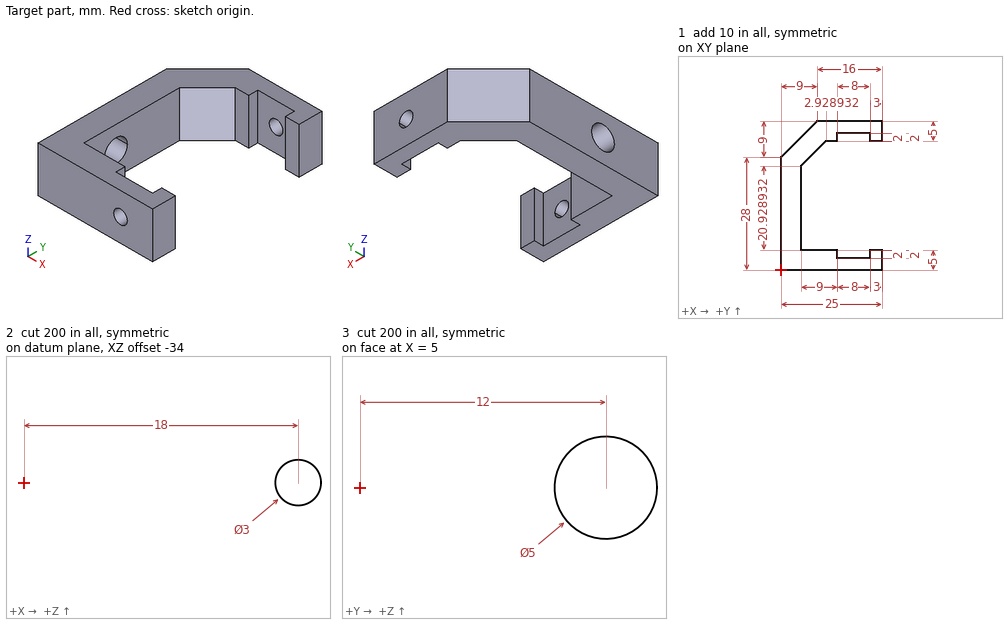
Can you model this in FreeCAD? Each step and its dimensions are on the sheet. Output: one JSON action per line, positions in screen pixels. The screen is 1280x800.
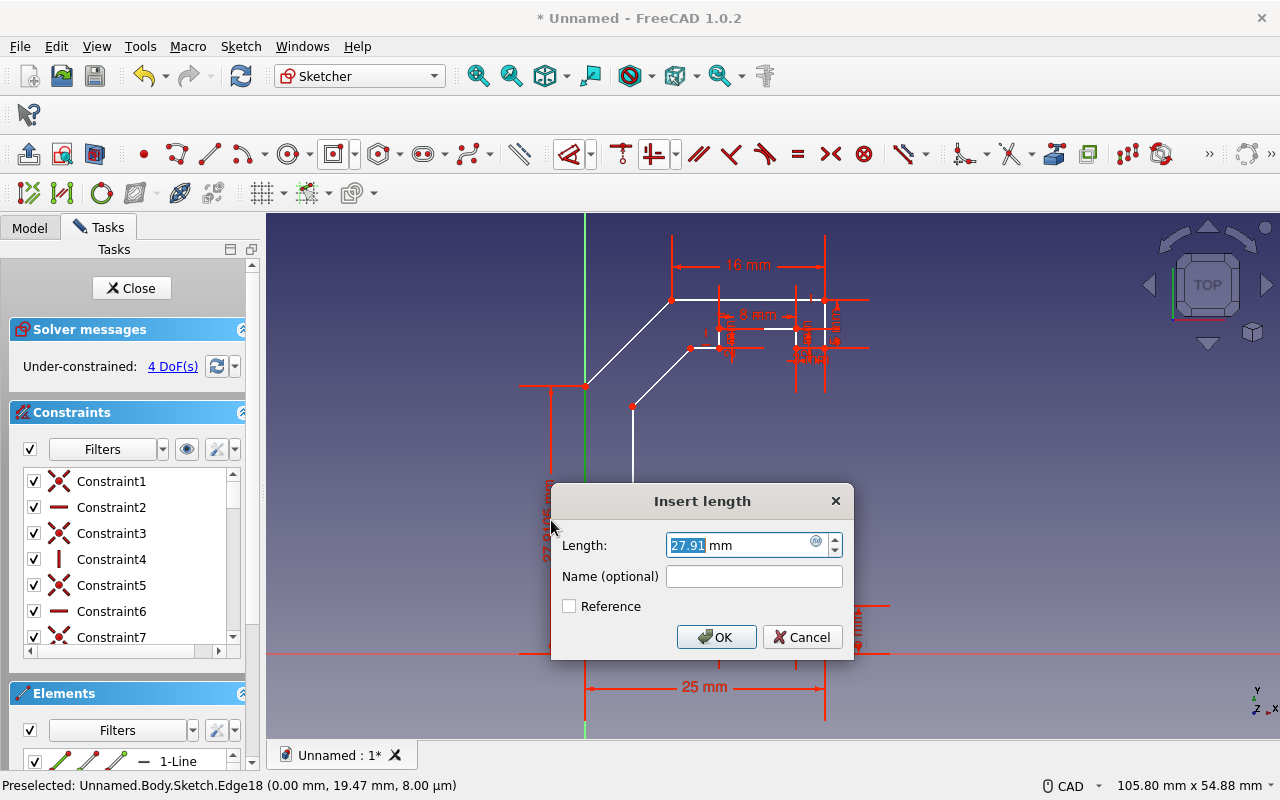
{"action": "type", "text": "28"}
{"action": "key", "text": "Return"}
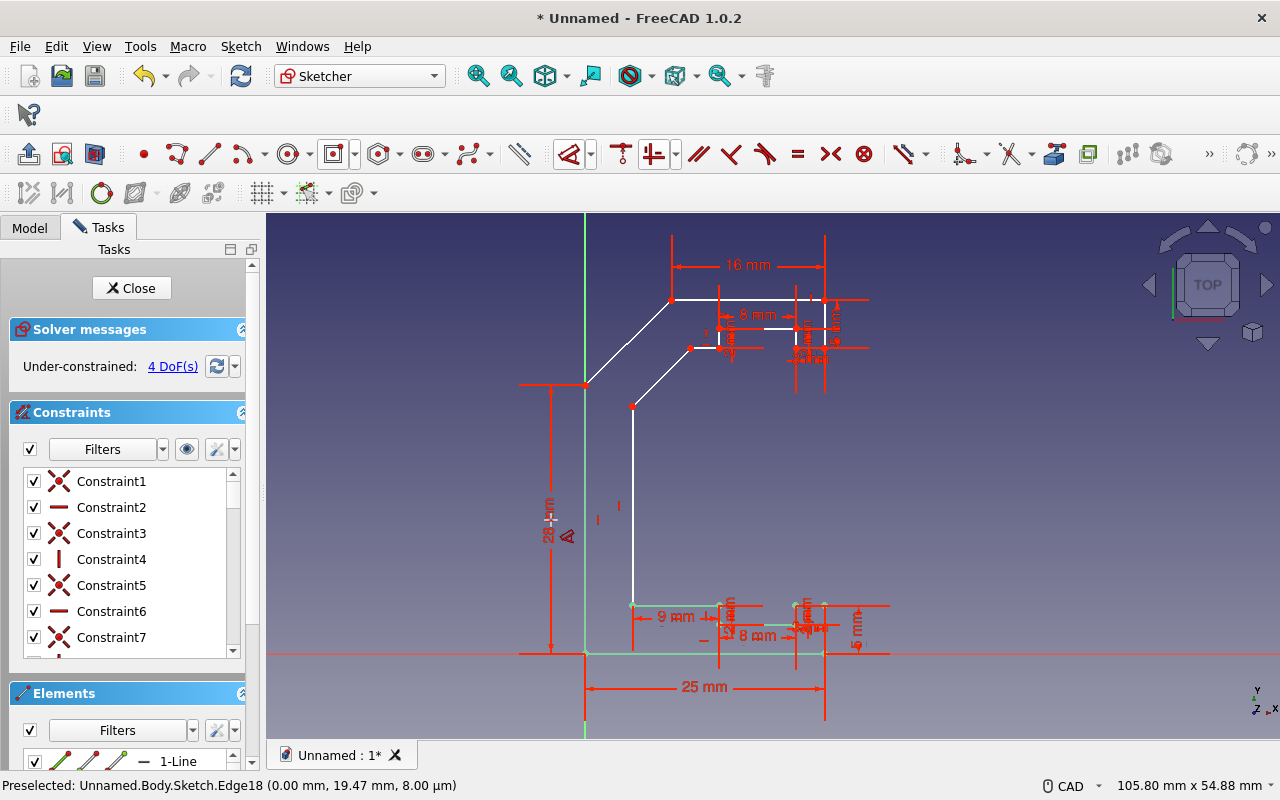
{"action": "left_click", "coordinate": [672, 300]}
{"action": "left_click", "coordinate": [628, 688]}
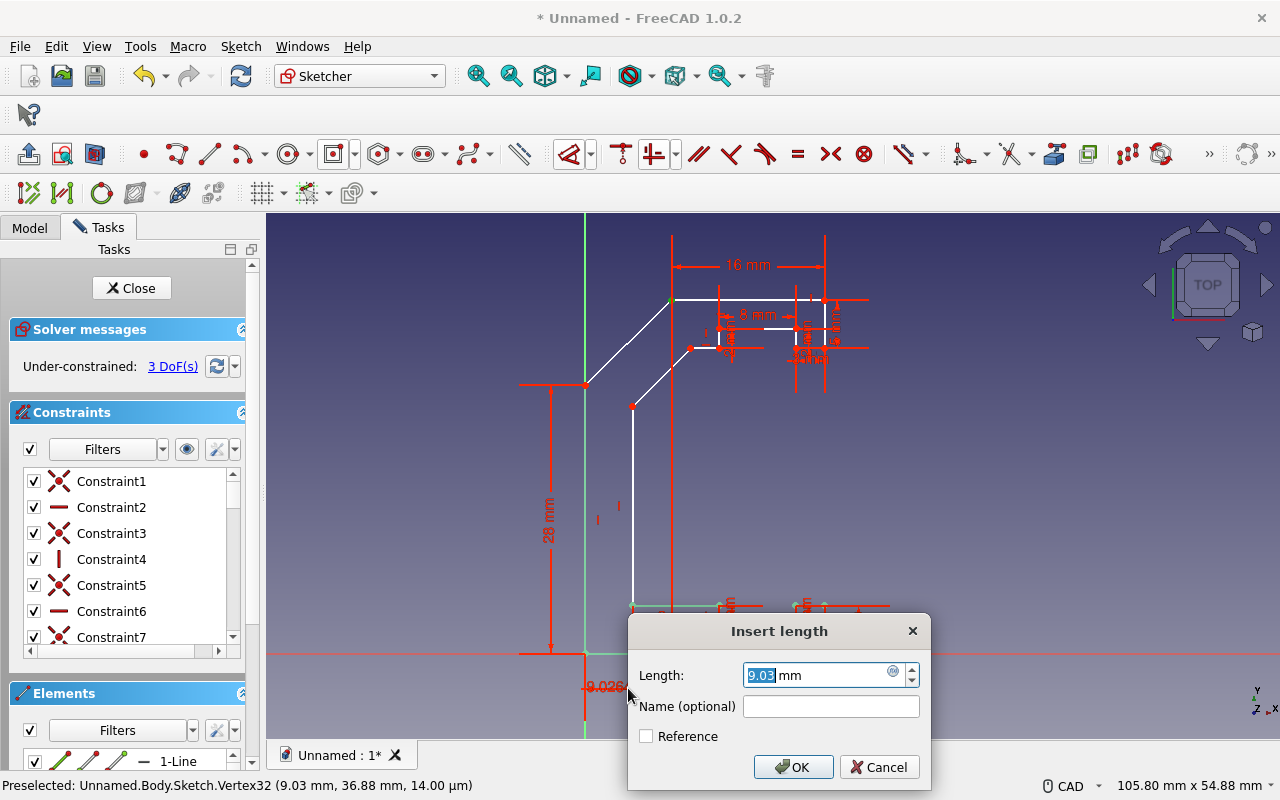
{"action": "type", "text": "9"}
{"action": "key", "text": "Return"}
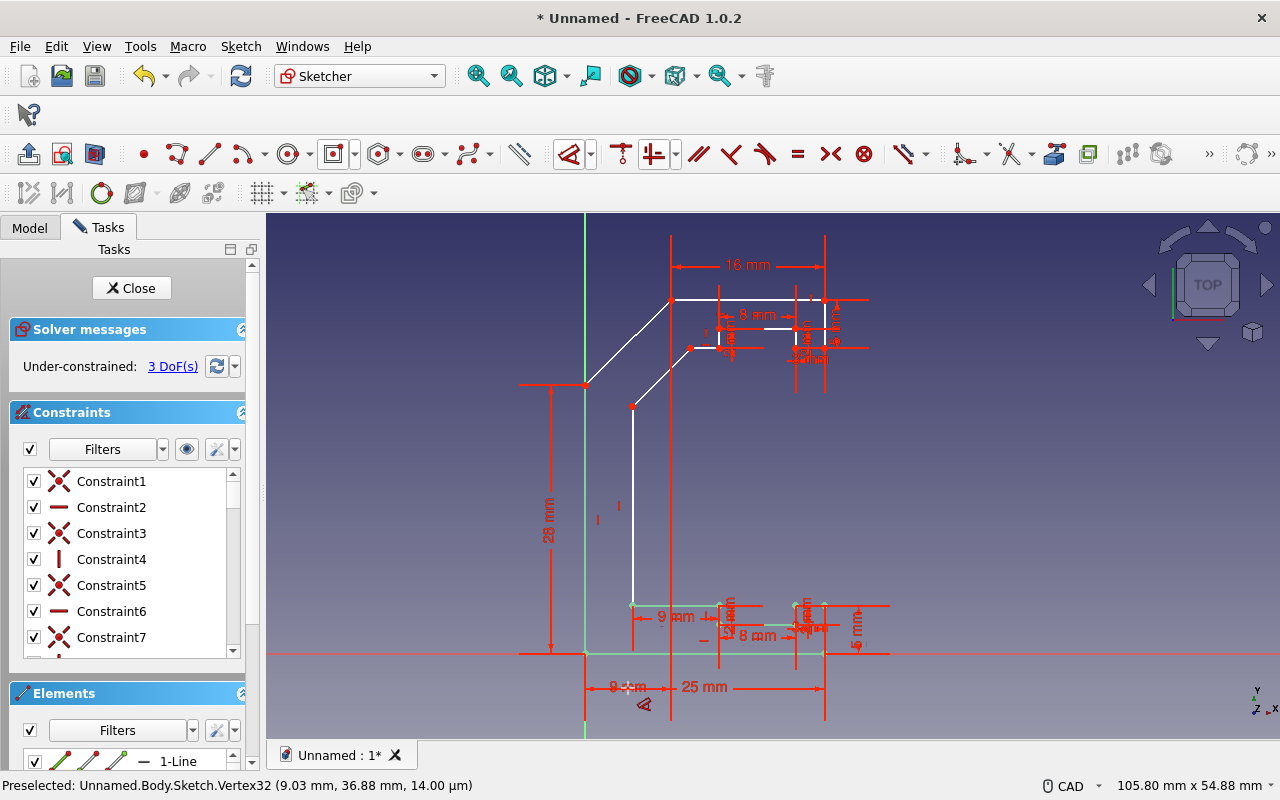
{"action": "left_click", "coordinate": [645, 326]}
{"action": "left_click", "coordinate": [551, 343]}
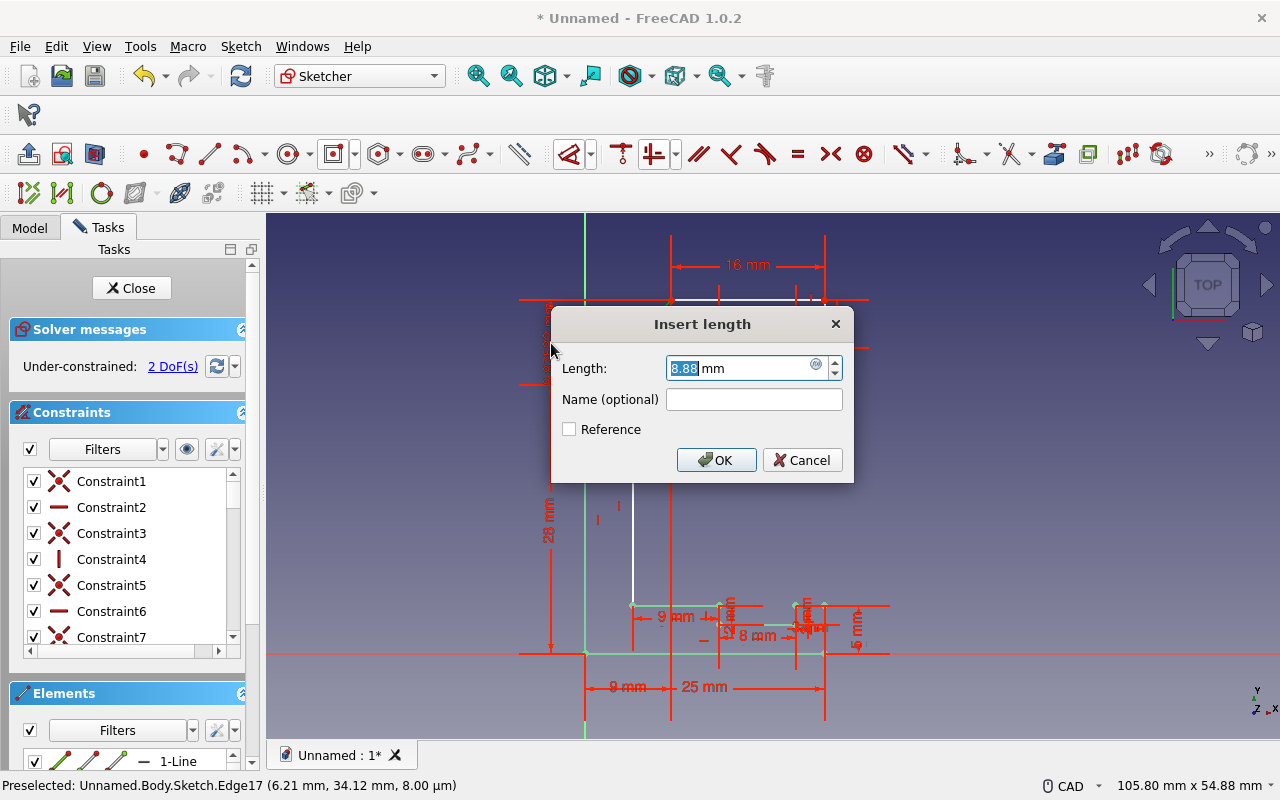
{"action": "type", "text": "9"}
{"action": "key", "text": "Return"}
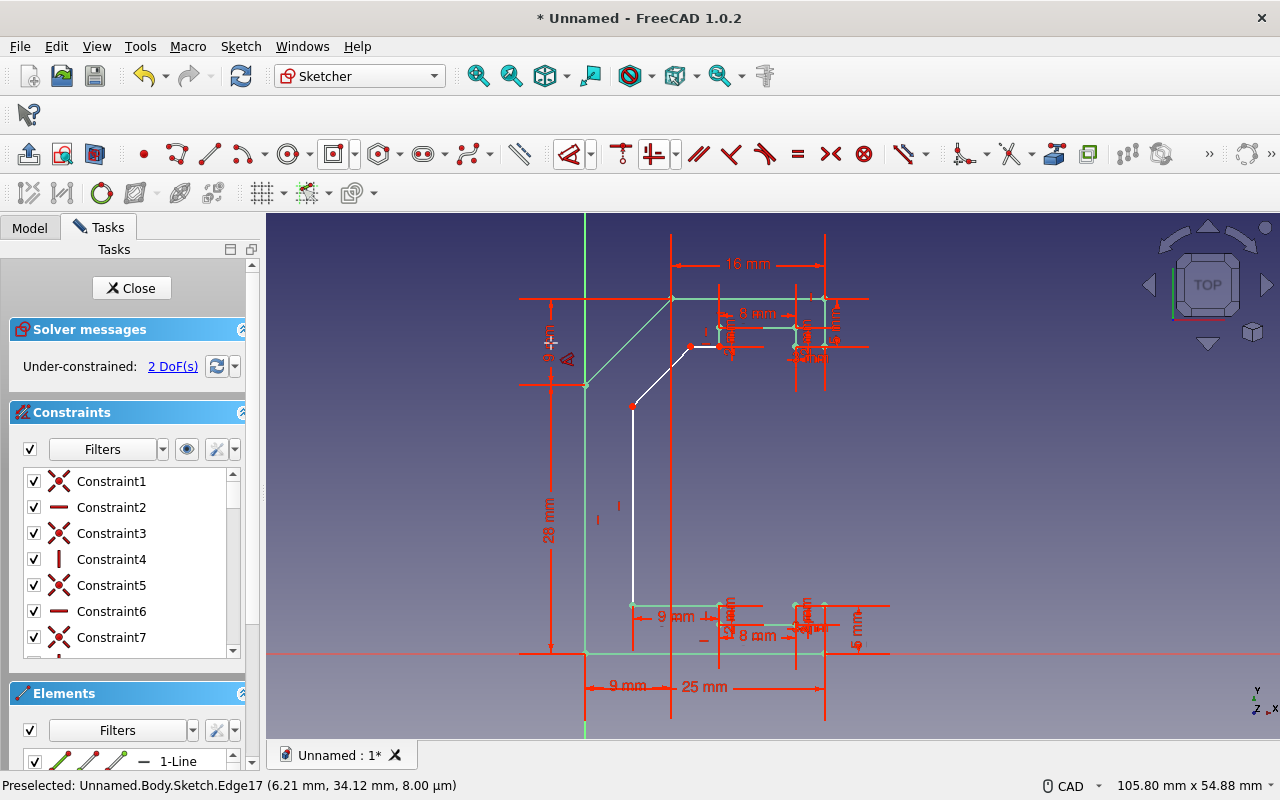
{"action": "scroll", "coordinate": [702, 347], "scroll_direction": "up", "scroll_amount": 2}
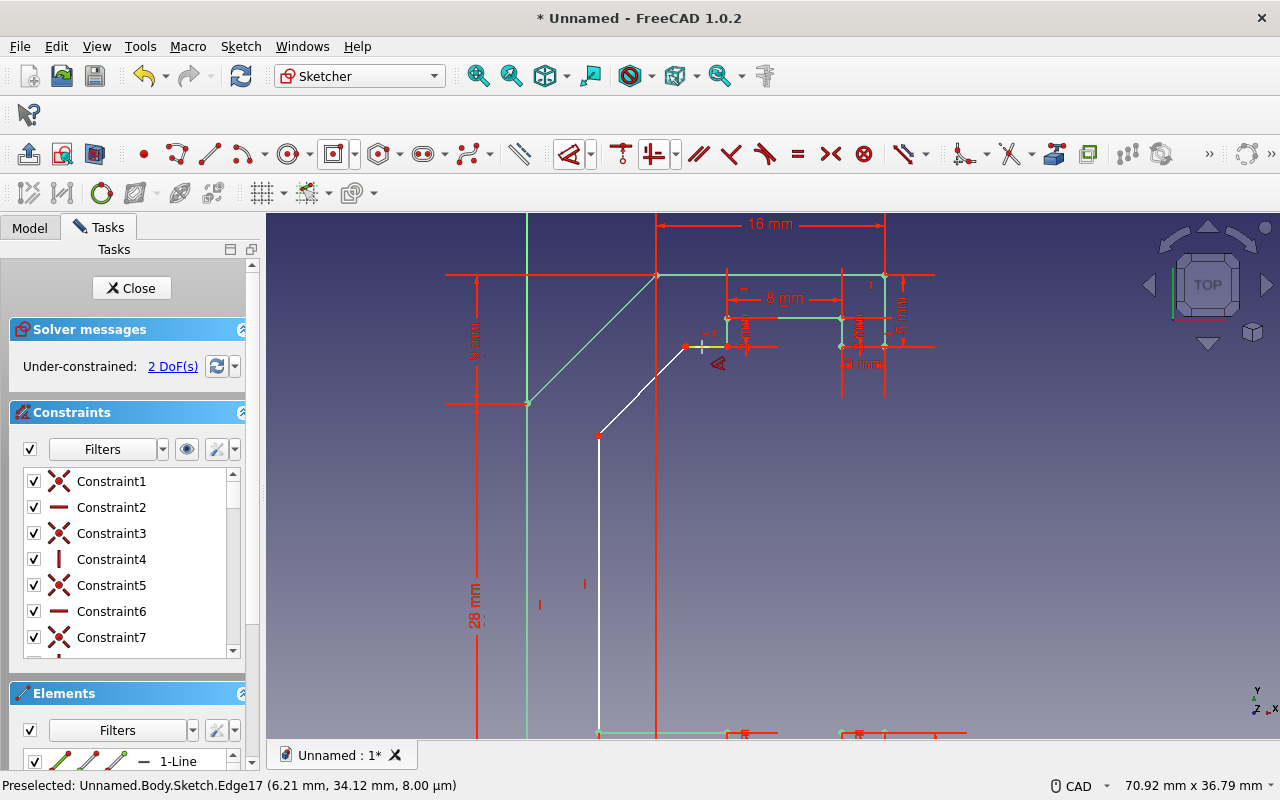
{"action": "left_click", "coordinate": [702, 347]}
{"action": "left_click", "coordinate": [706, 313]}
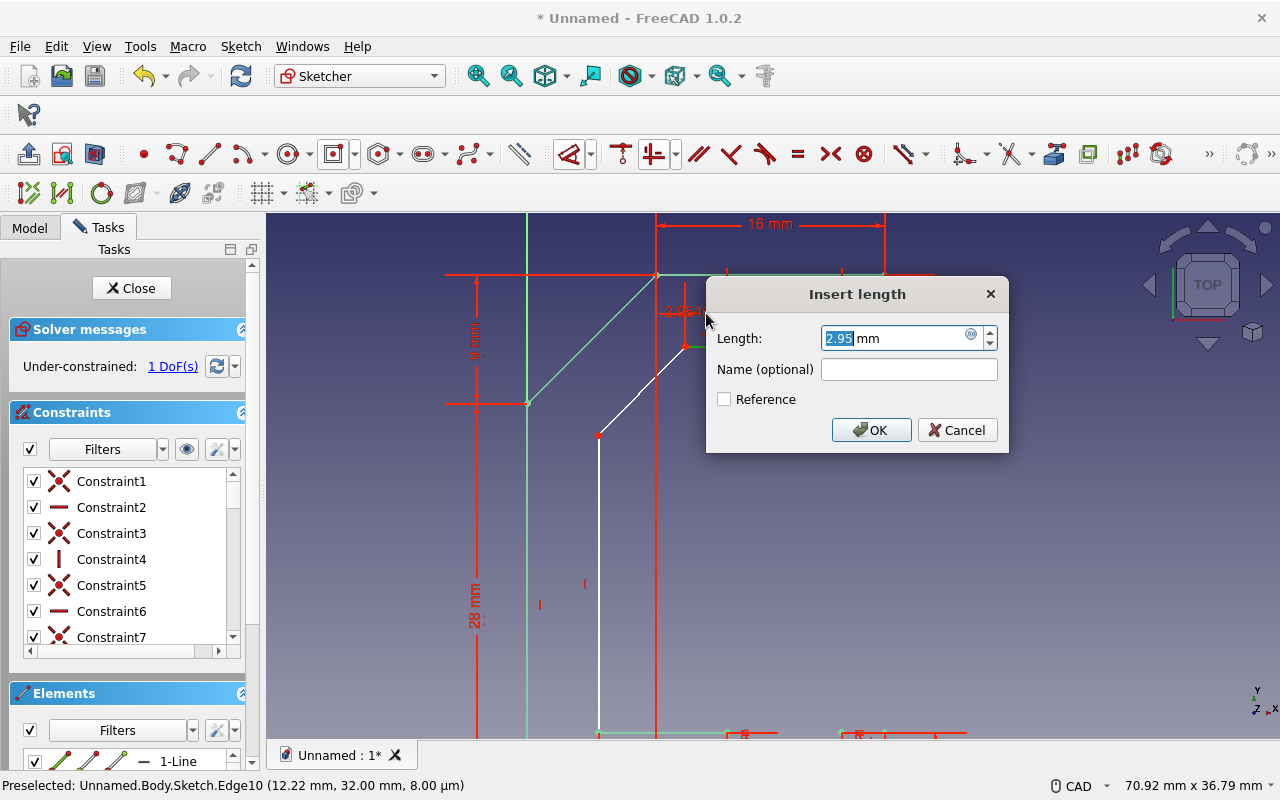
{"action": "type", "text": "2.928932"}
{"action": "key", "text": "Return"}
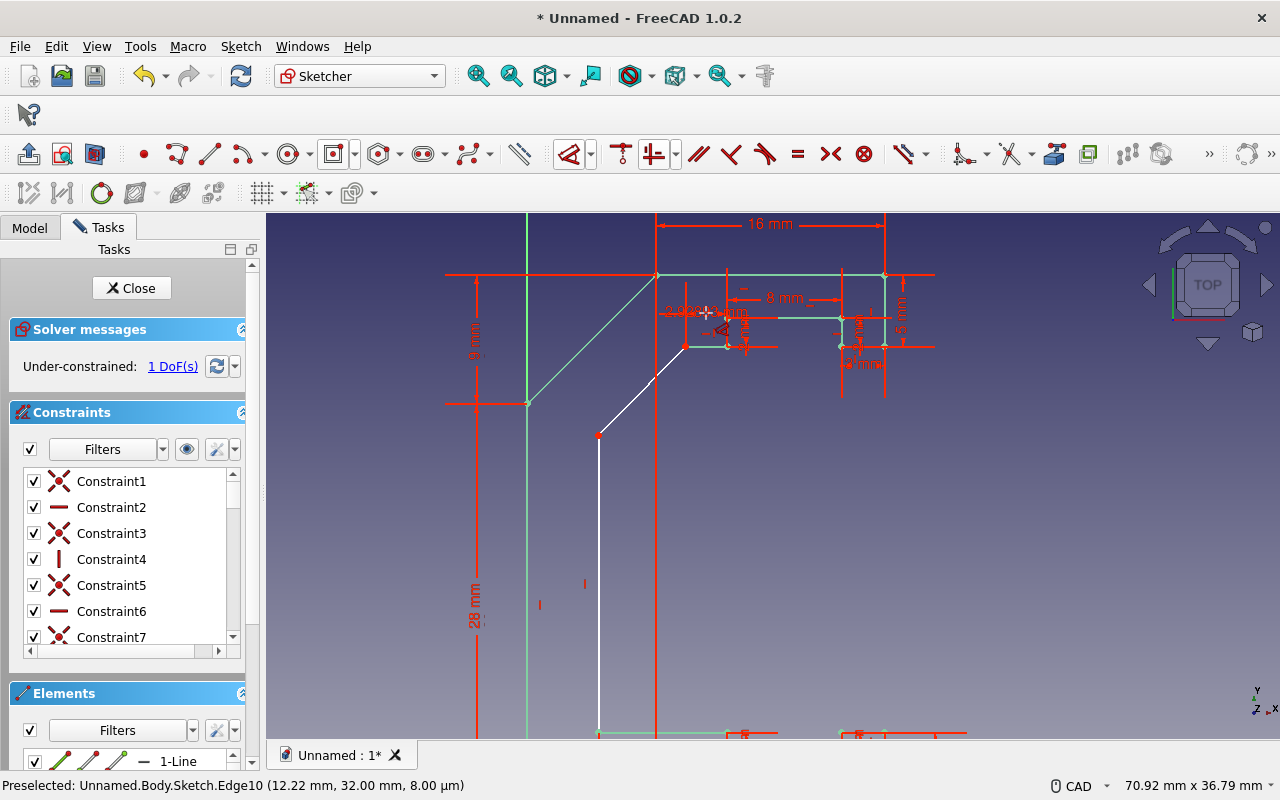
{"action": "left_click", "coordinate": [599, 643]}
{"action": "left_click", "coordinate": [565, 573]}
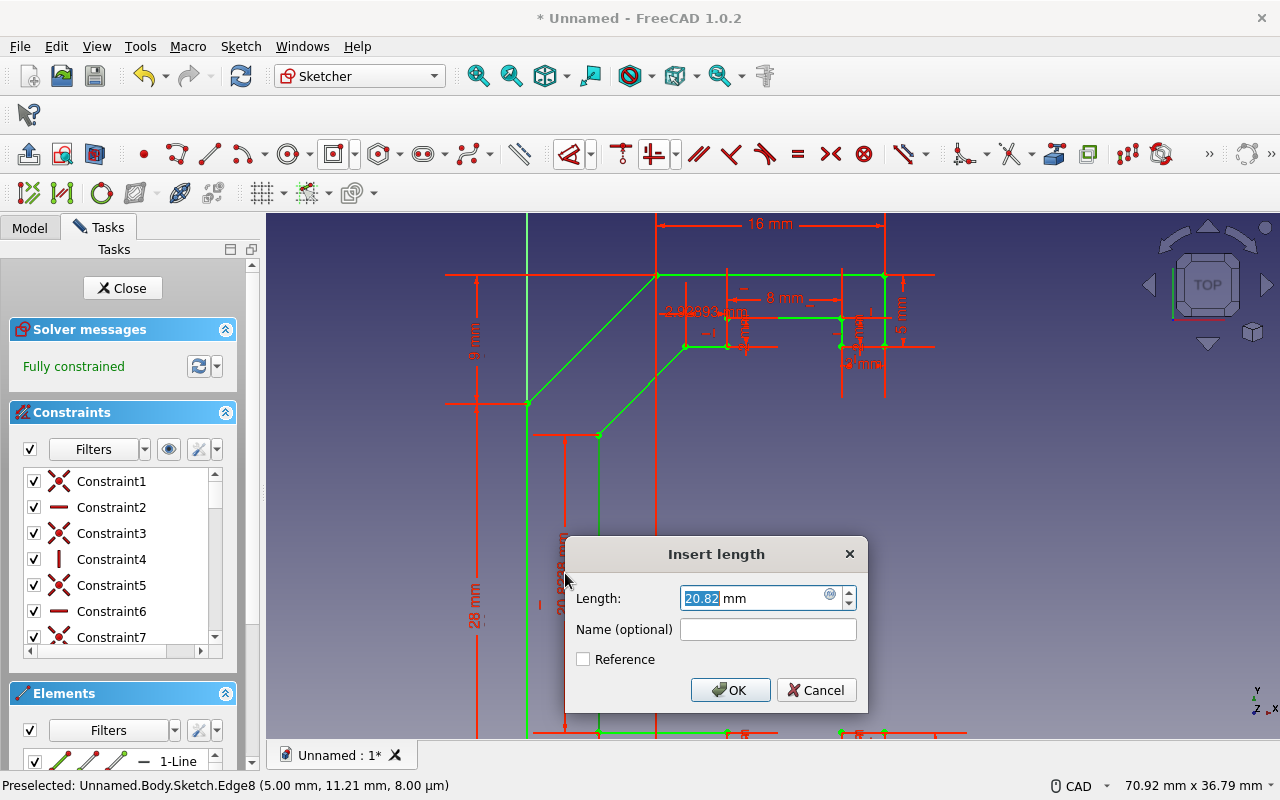
{"action": "type", "text": "20.928932"}
{"action": "key", "text": "Return"}
{"action": "key", "text": "Escape"}